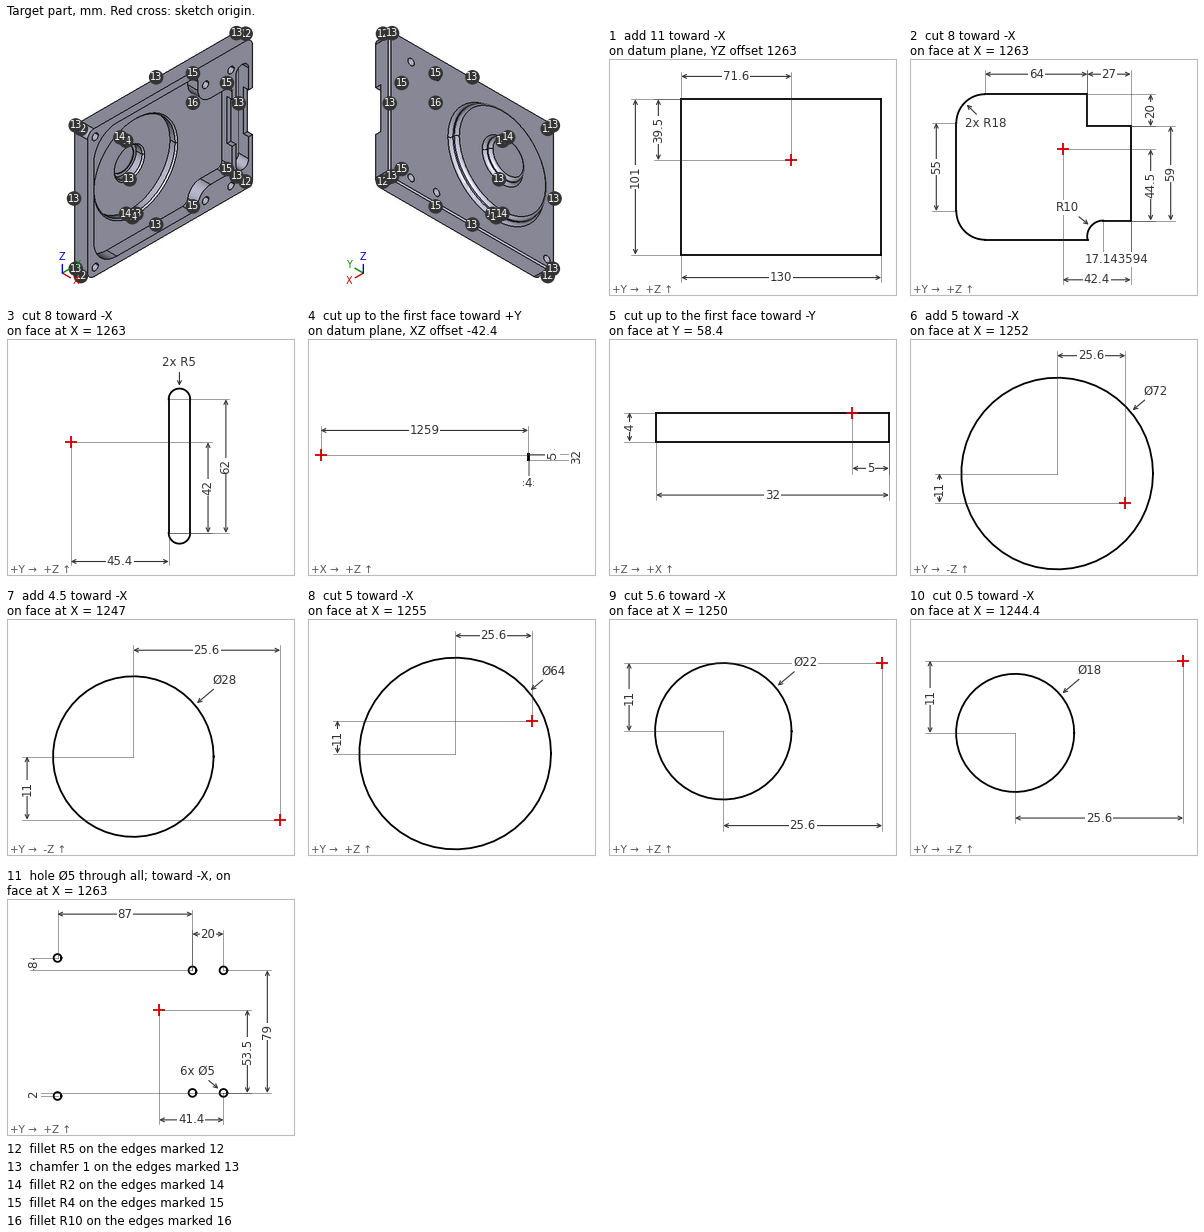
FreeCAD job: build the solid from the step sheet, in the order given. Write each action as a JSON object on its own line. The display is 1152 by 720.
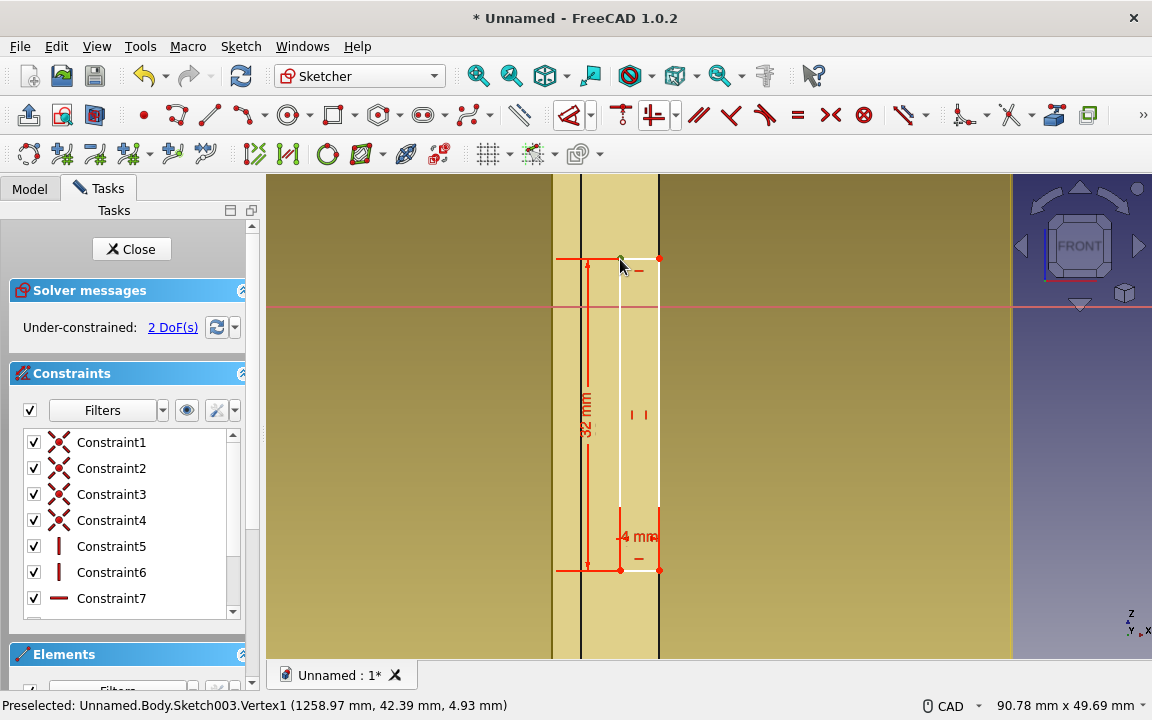
{"action": "key", "text": "i"}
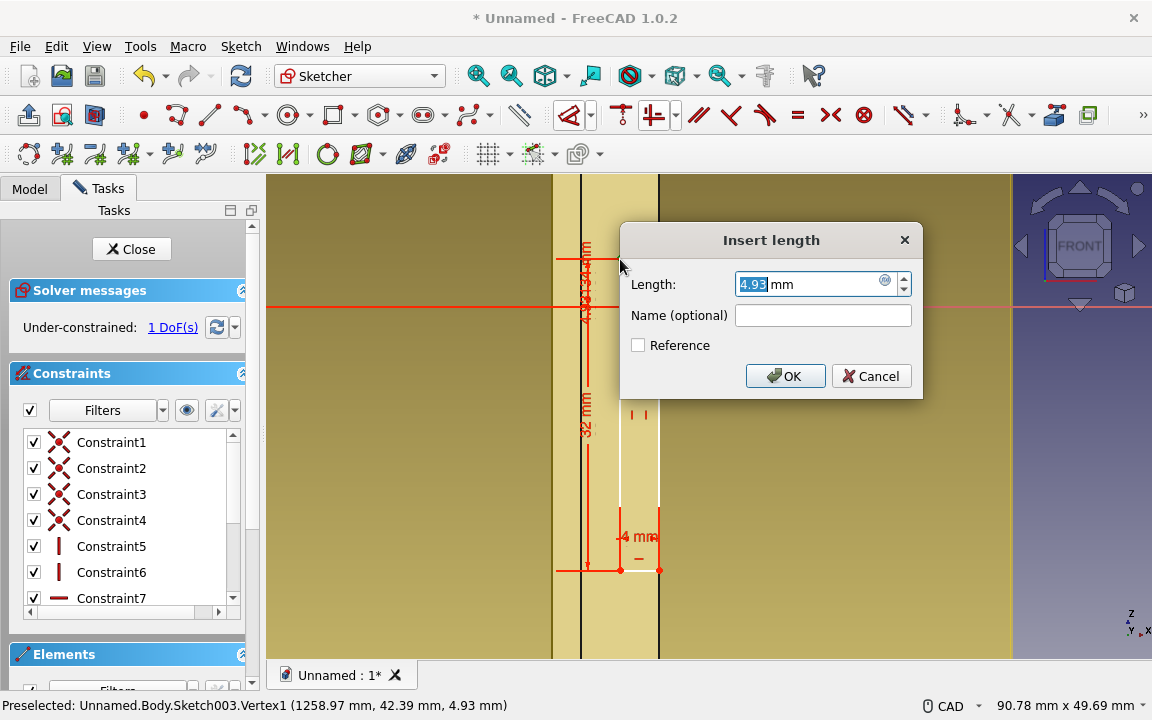
{"action": "type", "text": "5"}
{"action": "key", "text": "Return"}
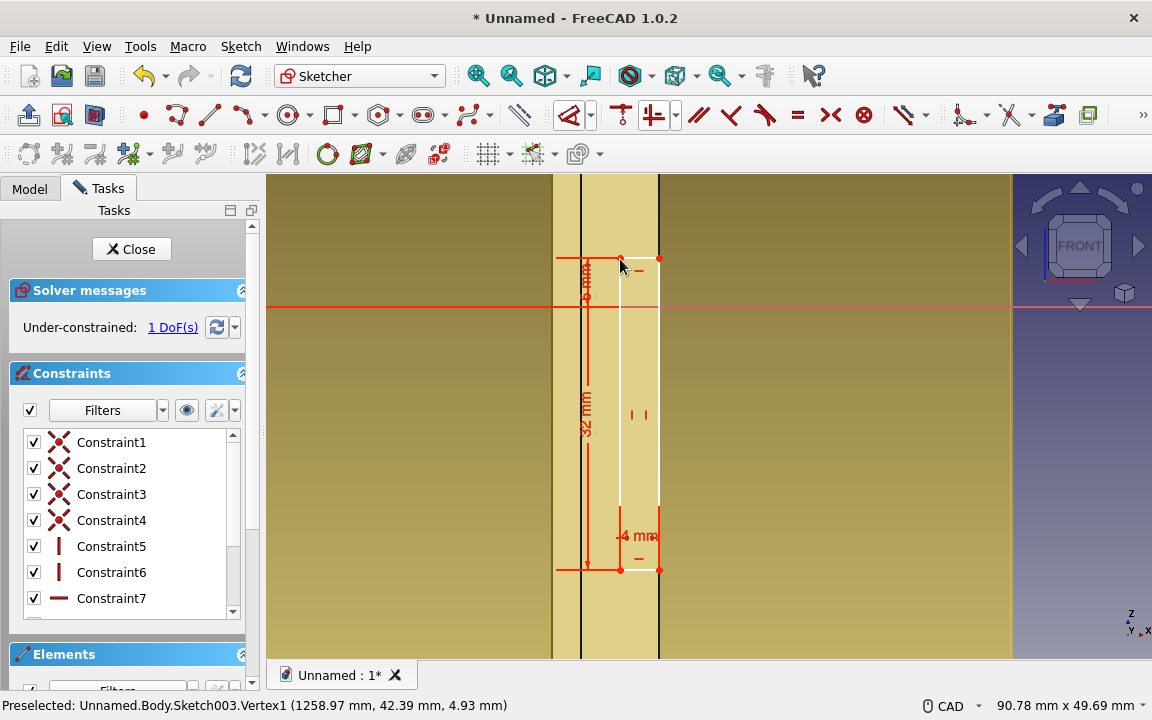
{"action": "left_click", "coordinate": [620, 258]}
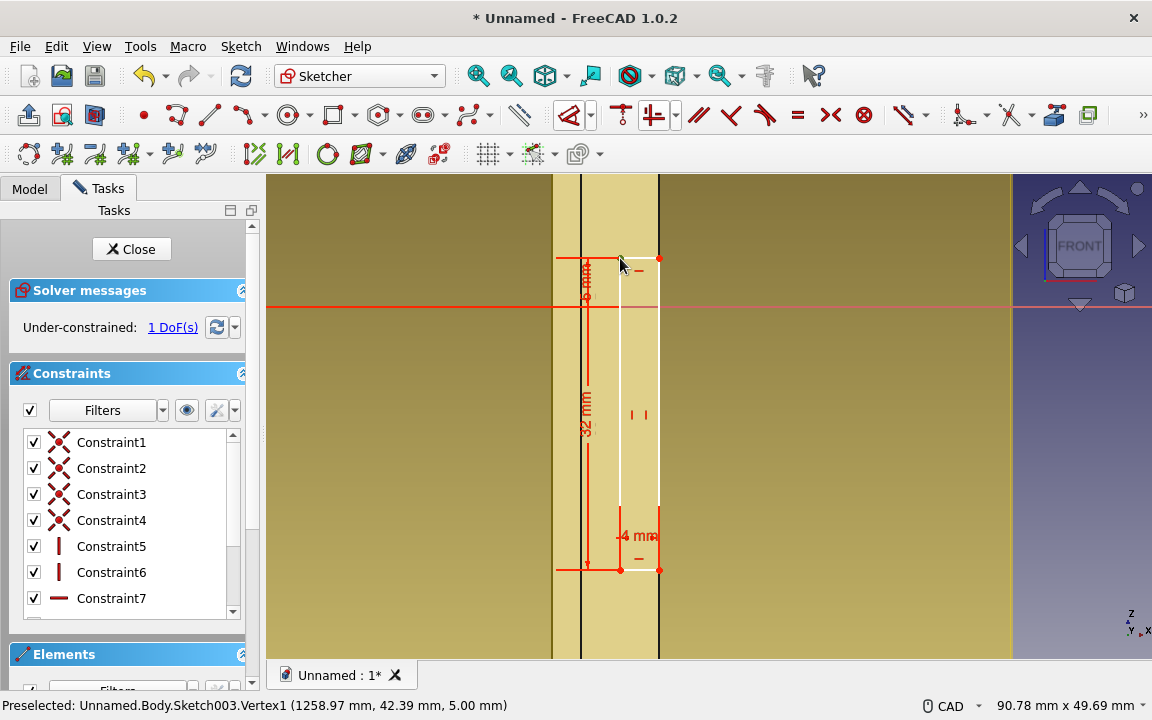
{"action": "left_click", "coordinate": [590, 116]}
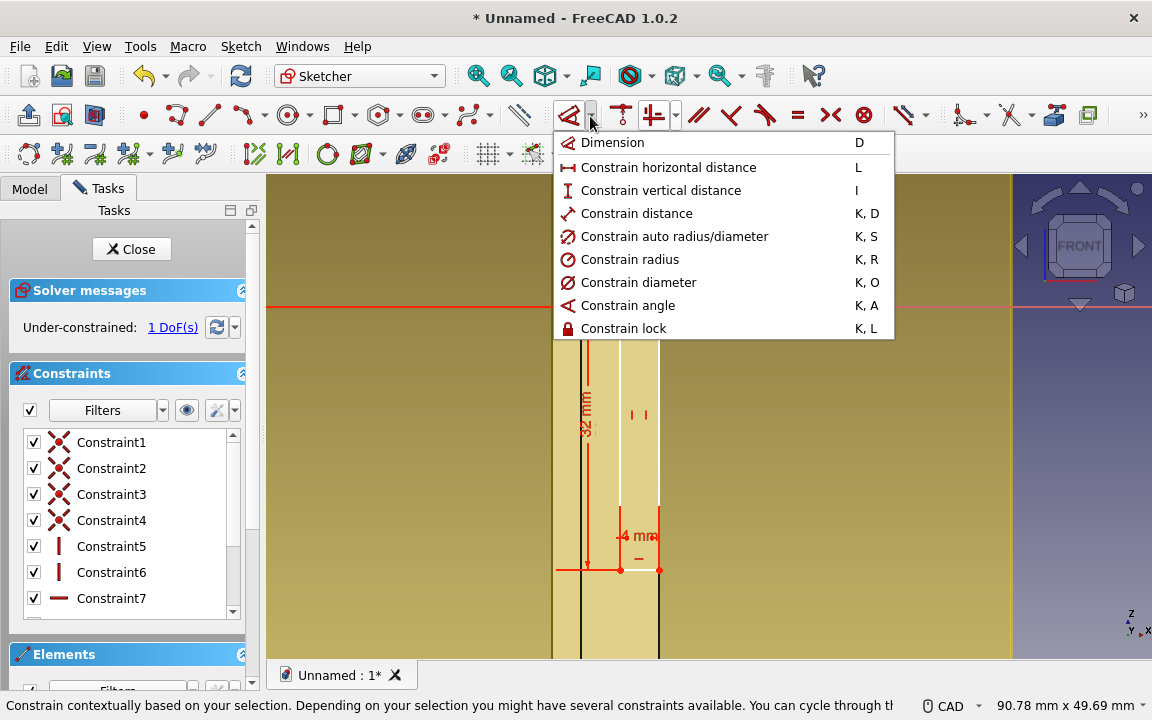
{"action": "left_click", "coordinate": [724, 168]}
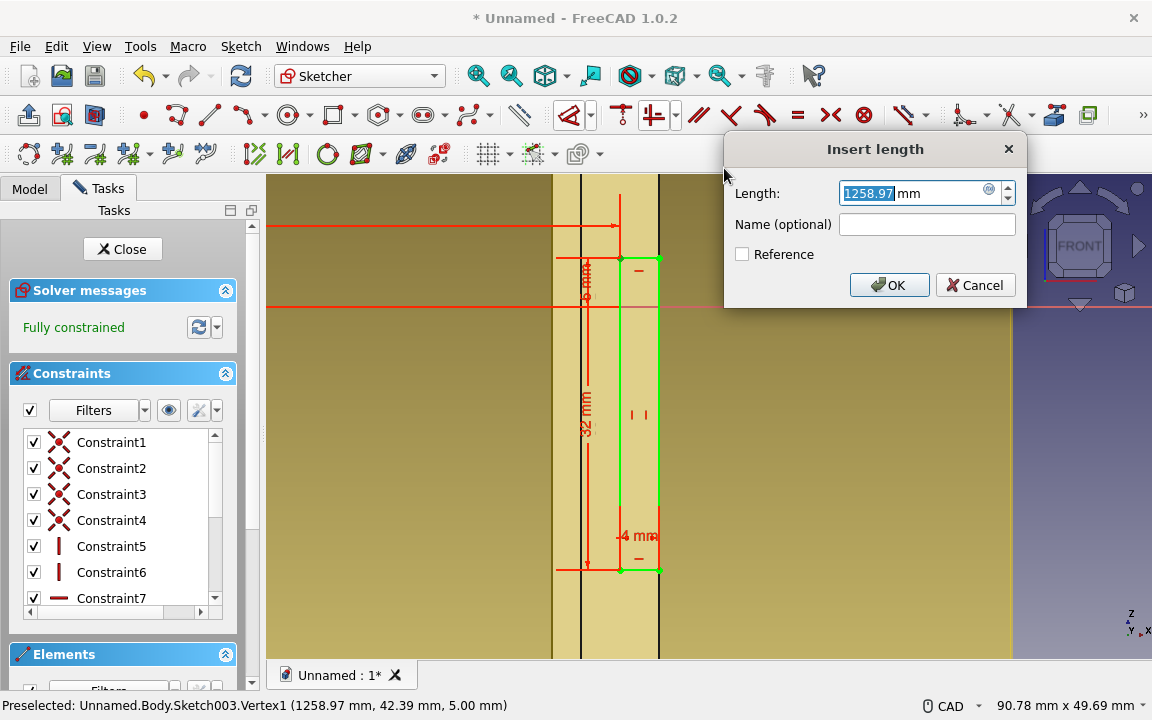
{"action": "type", "text": "1259"}
{"action": "key", "text": "Return"}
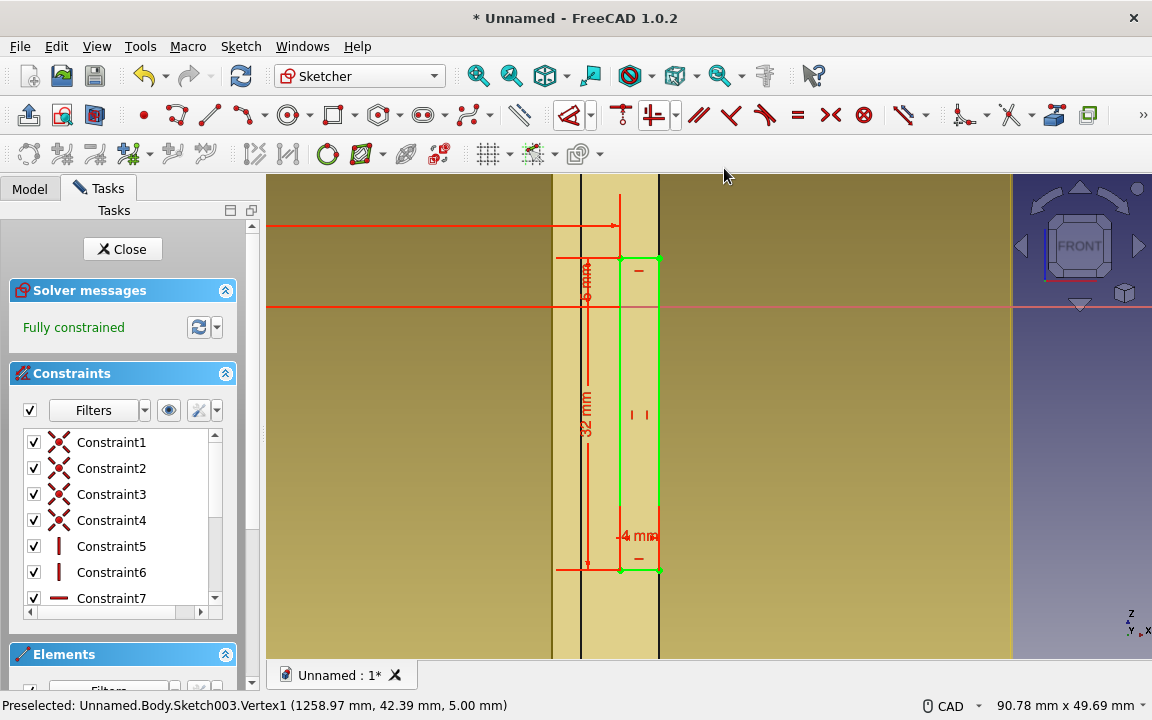
{"action": "left_click", "coordinate": [123, 249]}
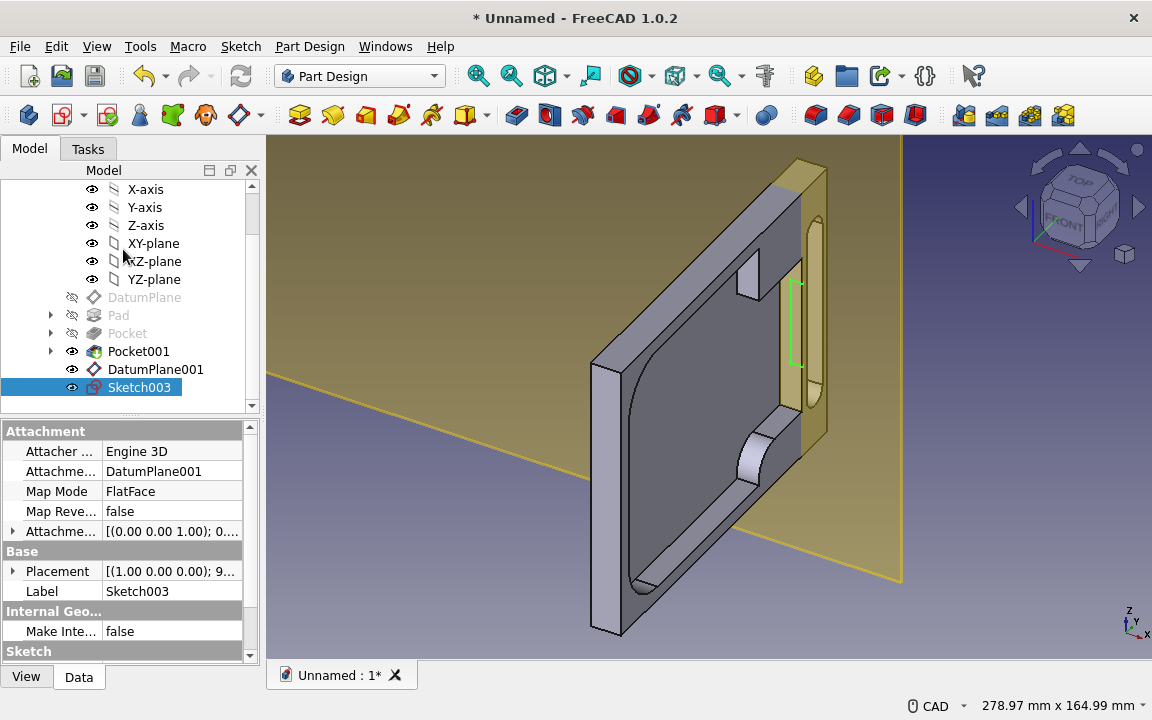
{"action": "left_click", "coordinate": [517, 116]}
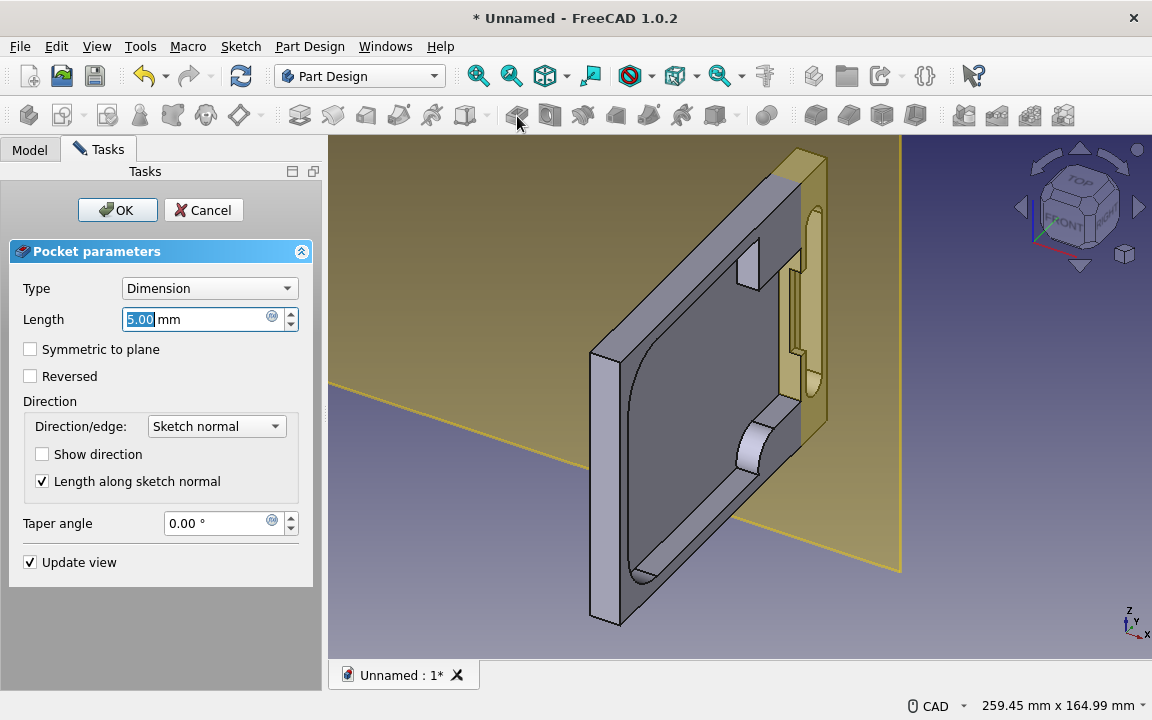
{"action": "left_click", "coordinate": [210, 288]}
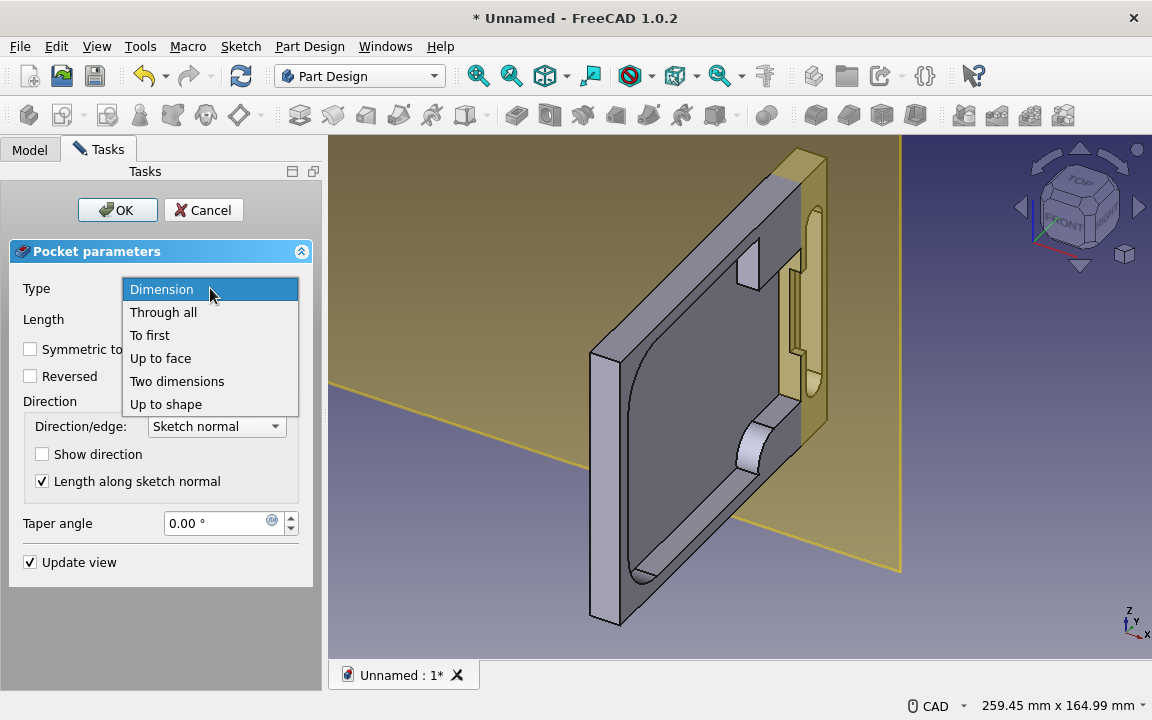
{"action": "left_click", "coordinate": [208, 336]}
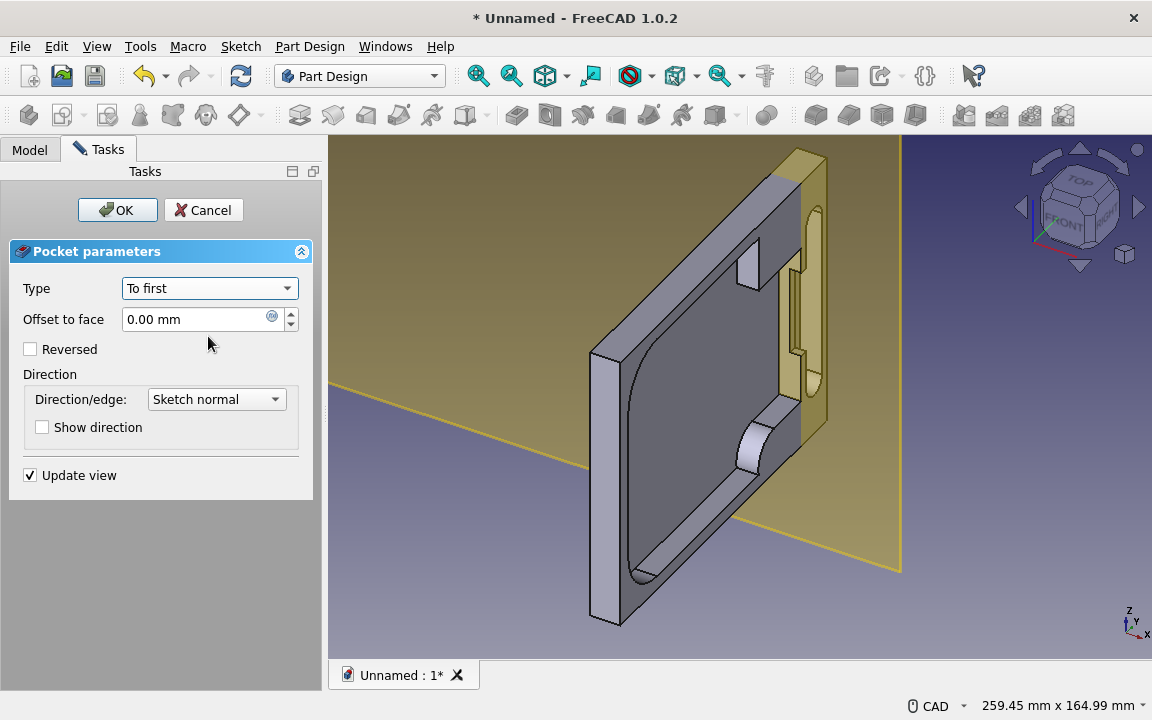
{"action": "left_click", "coordinate": [118, 210]}